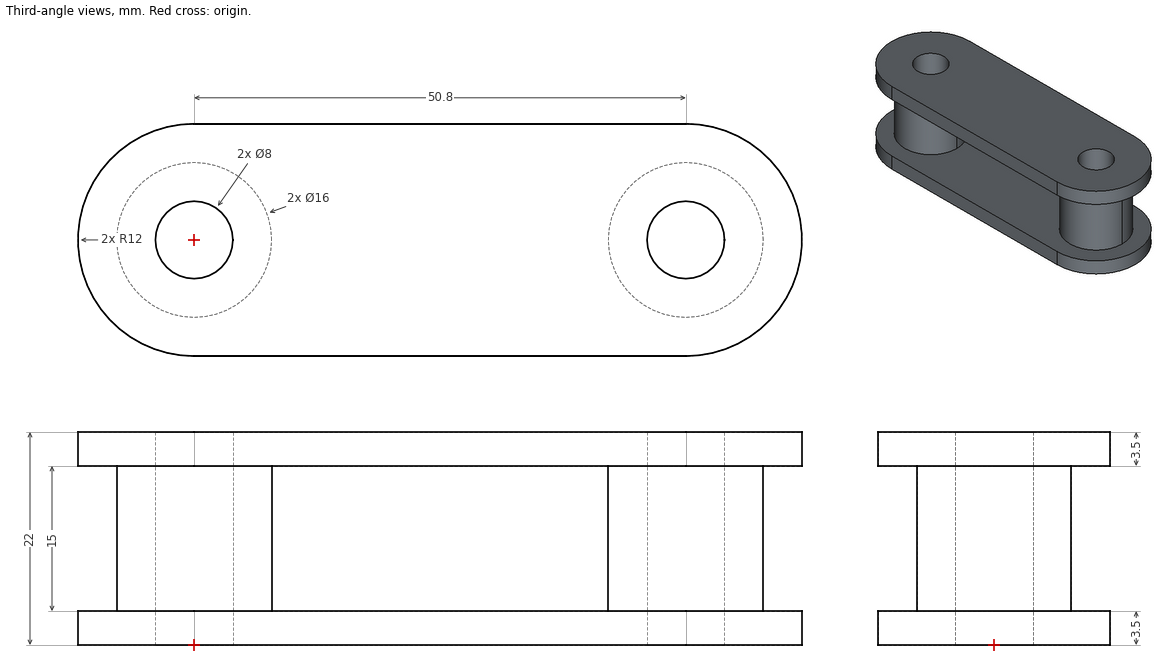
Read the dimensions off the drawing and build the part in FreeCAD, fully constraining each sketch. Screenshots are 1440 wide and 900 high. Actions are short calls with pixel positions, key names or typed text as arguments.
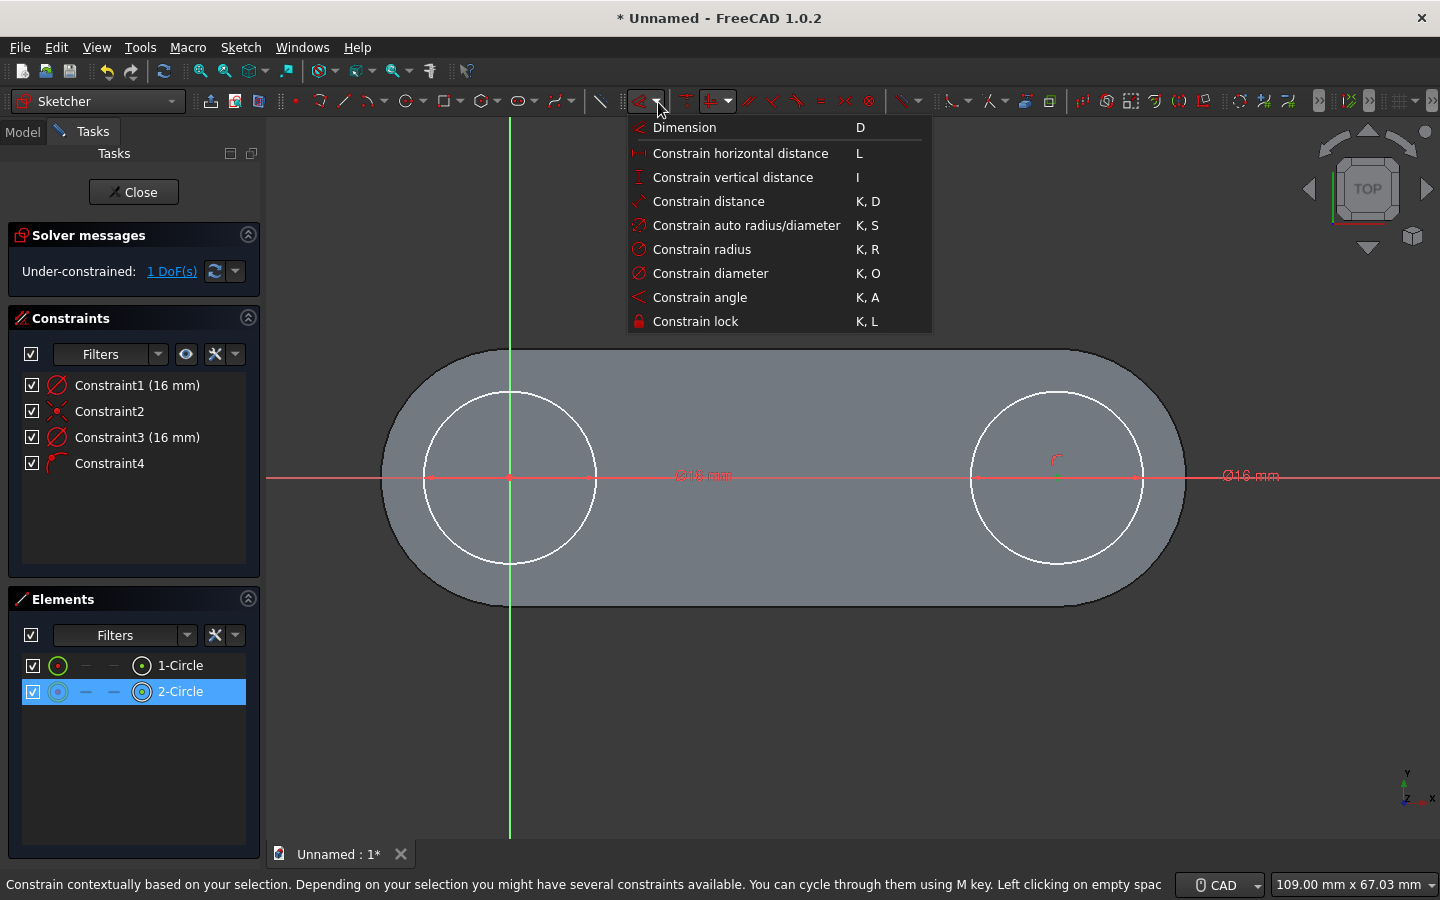
click(780, 153)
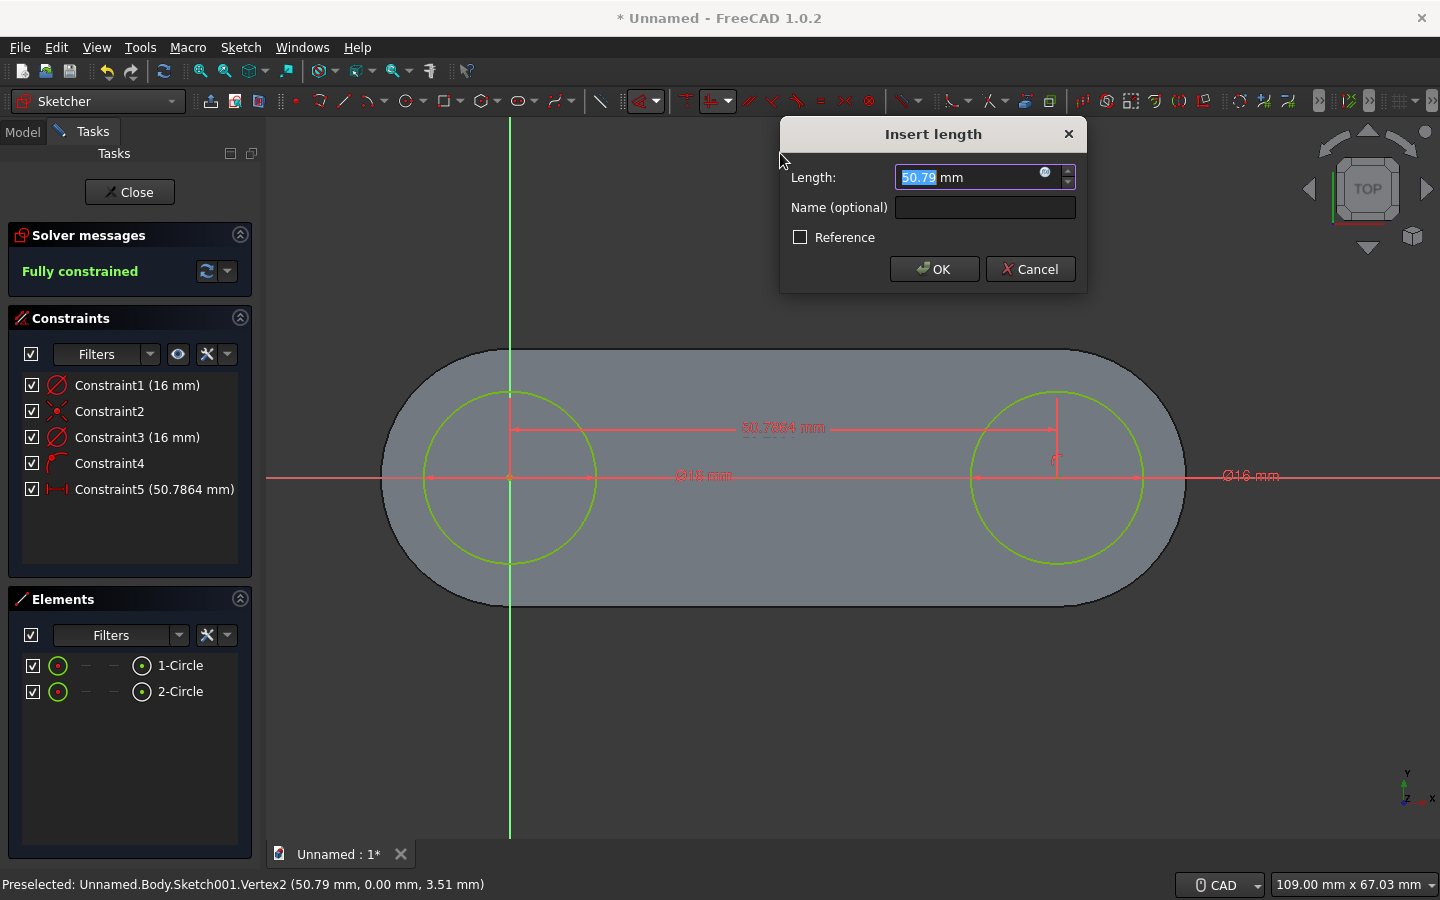
text(50.8)
key(Return)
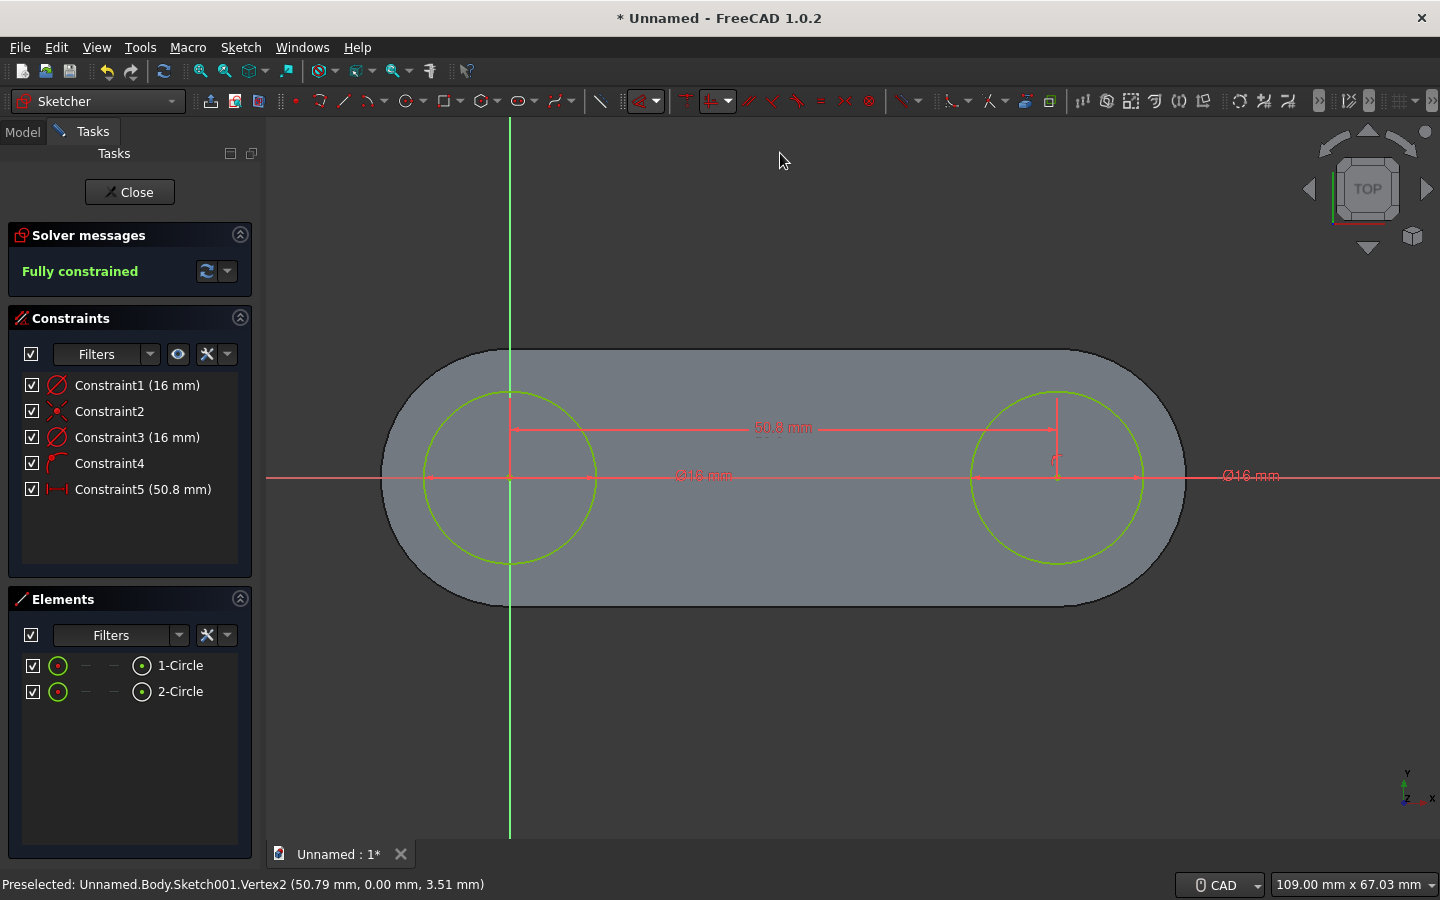
click(130, 192)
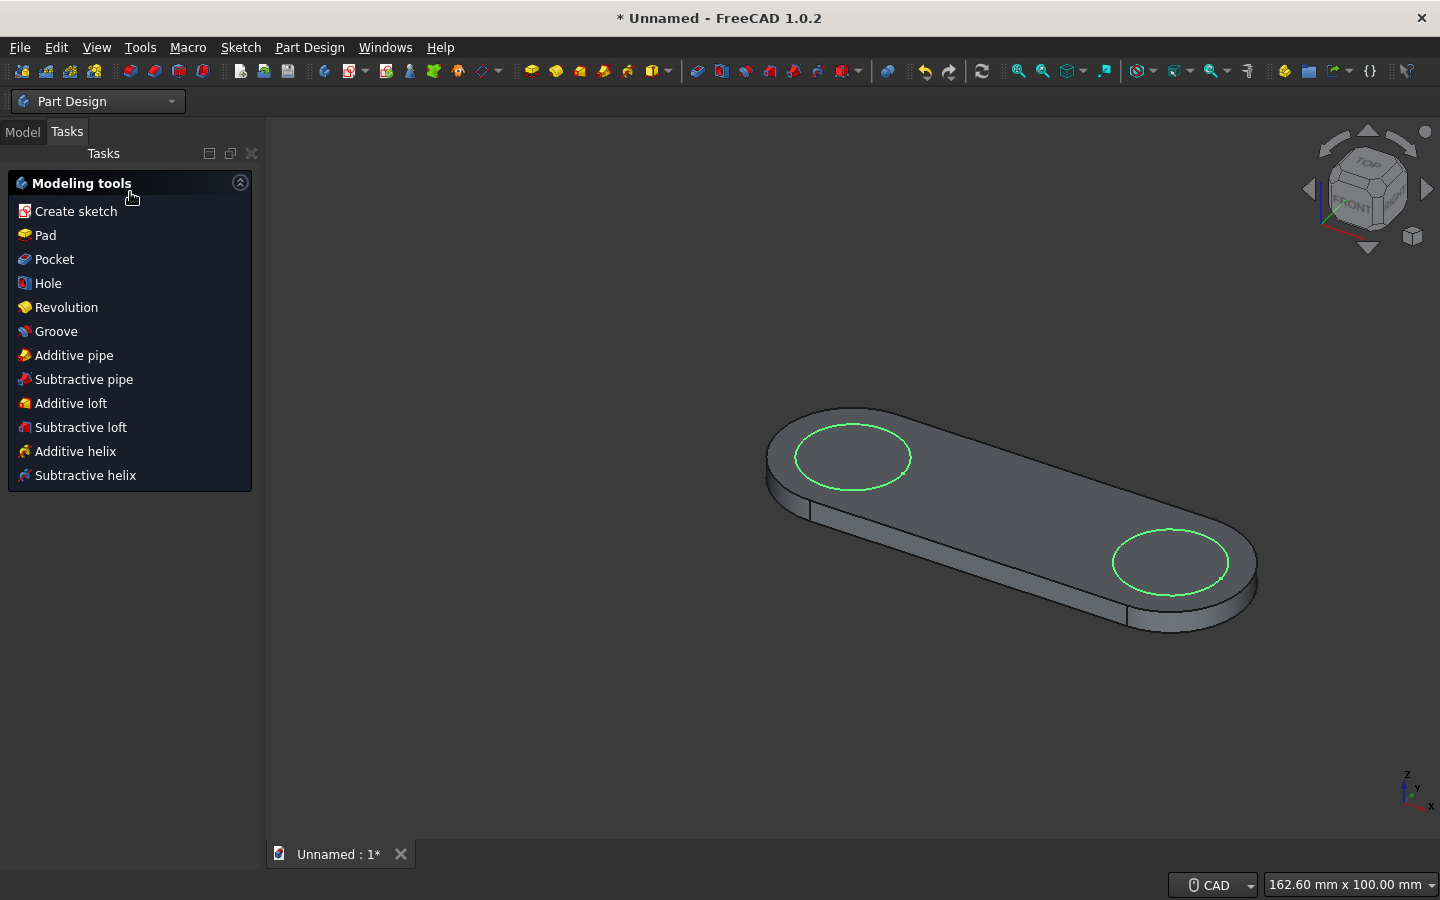
click(532, 72)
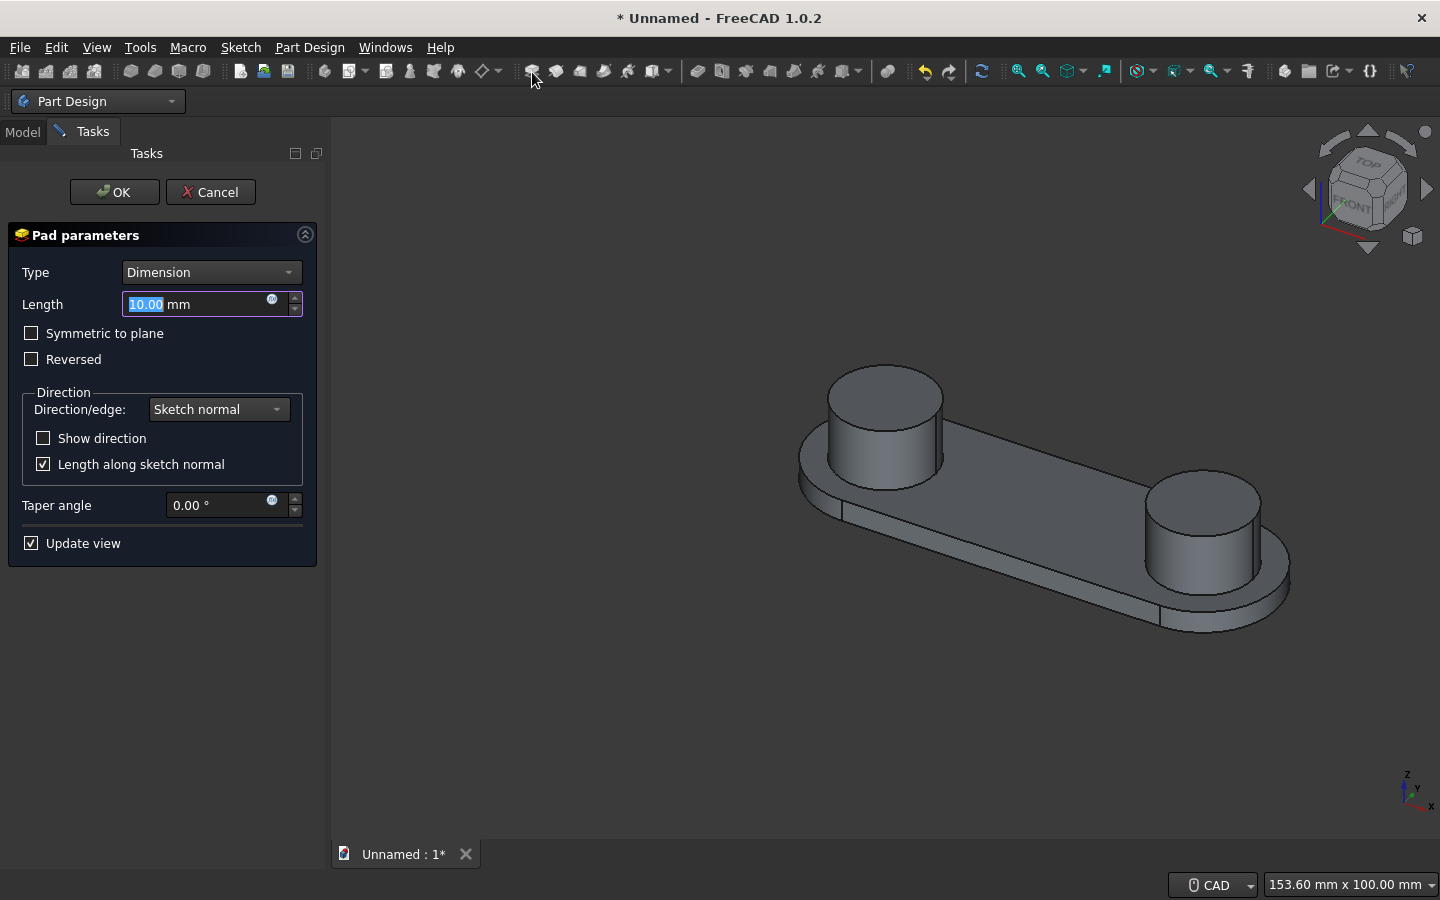
text(15)
key(Tab)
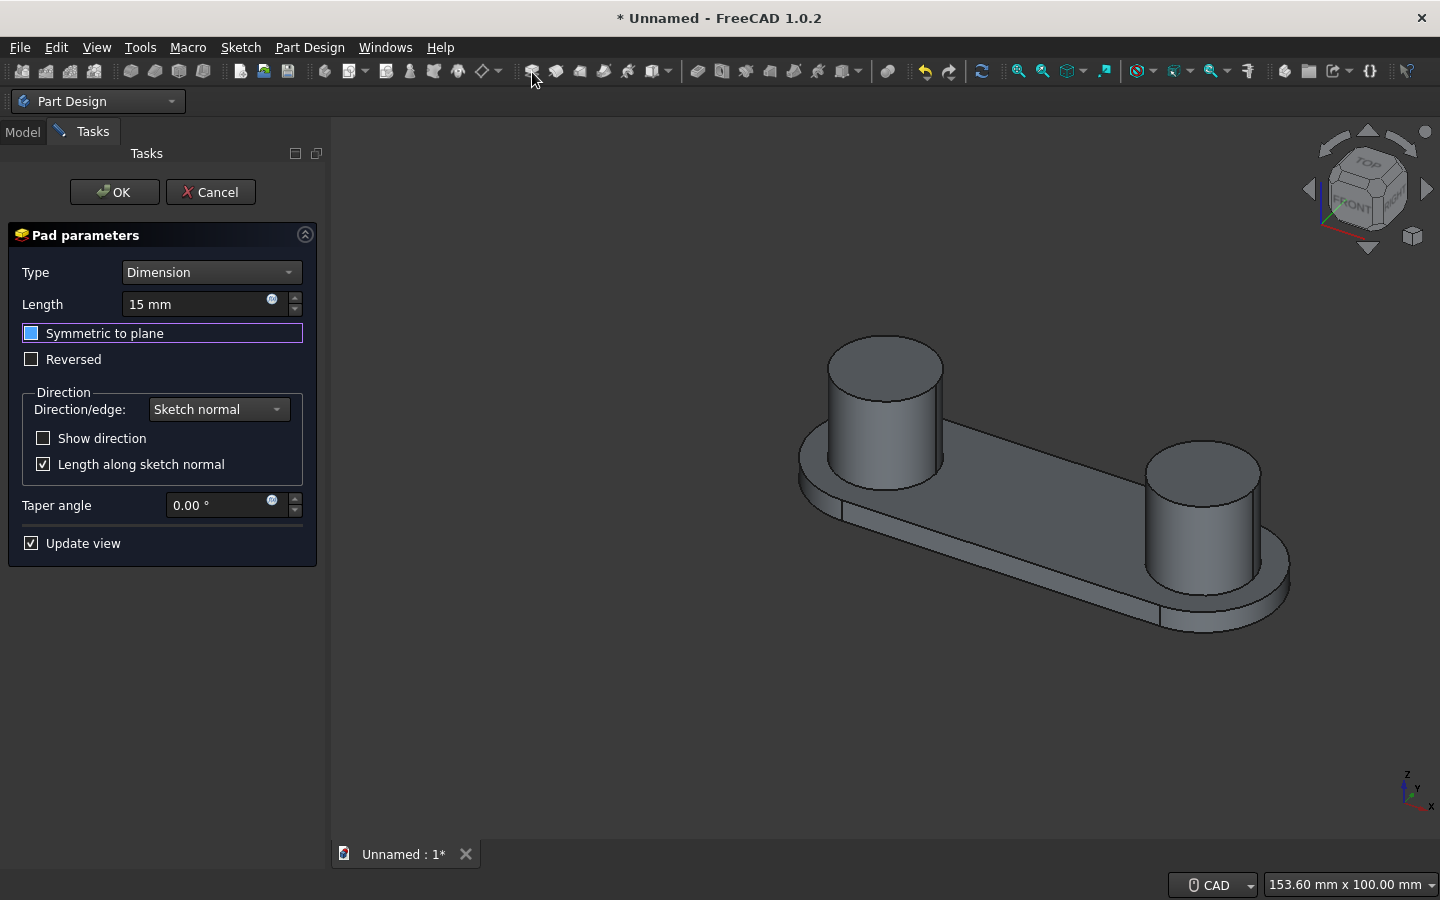
click(115, 192)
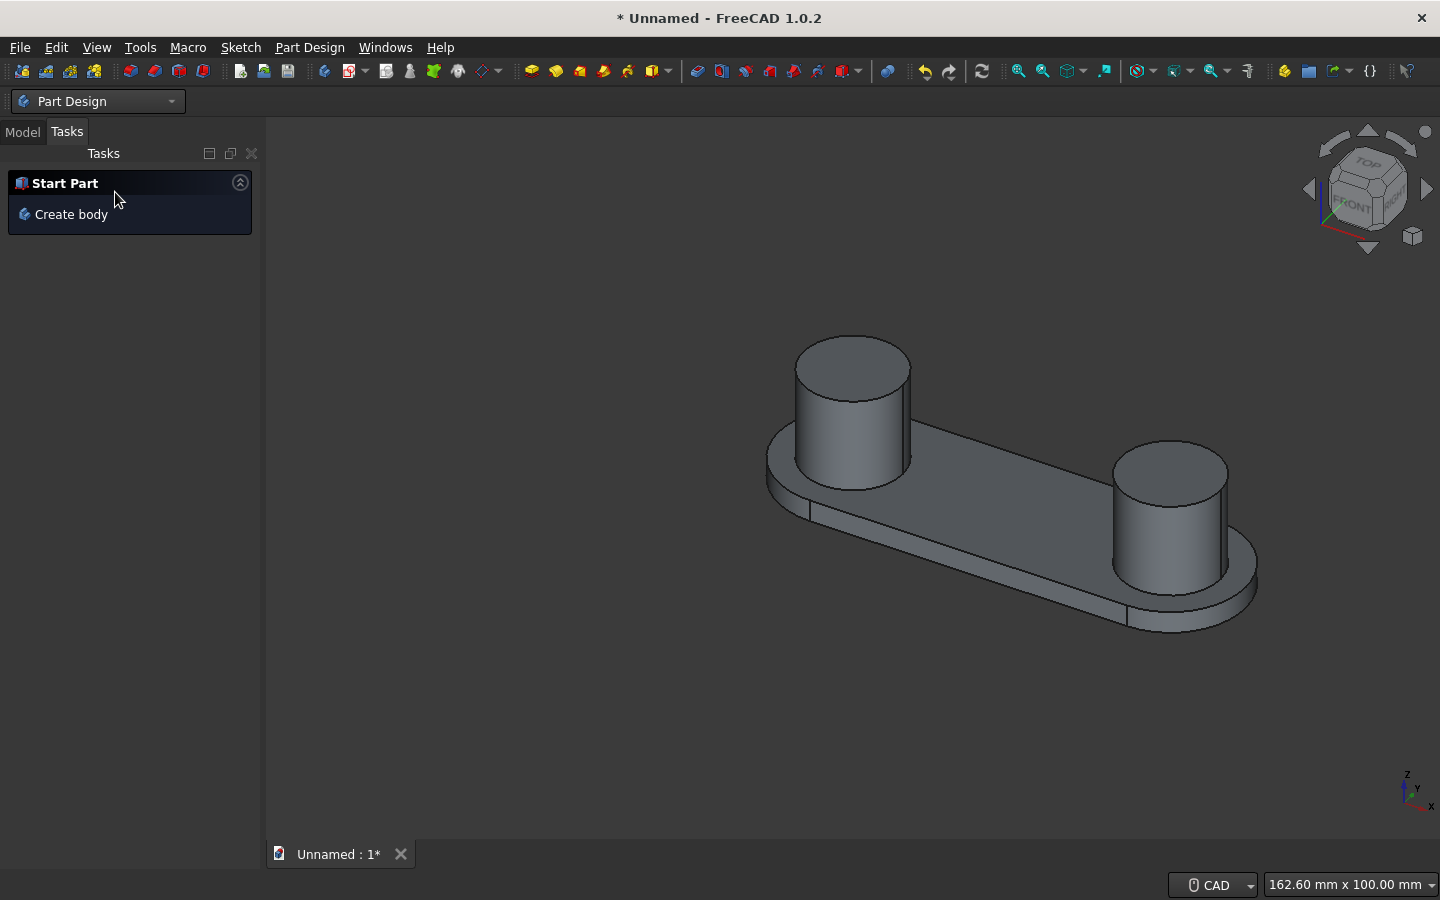
click(853, 368)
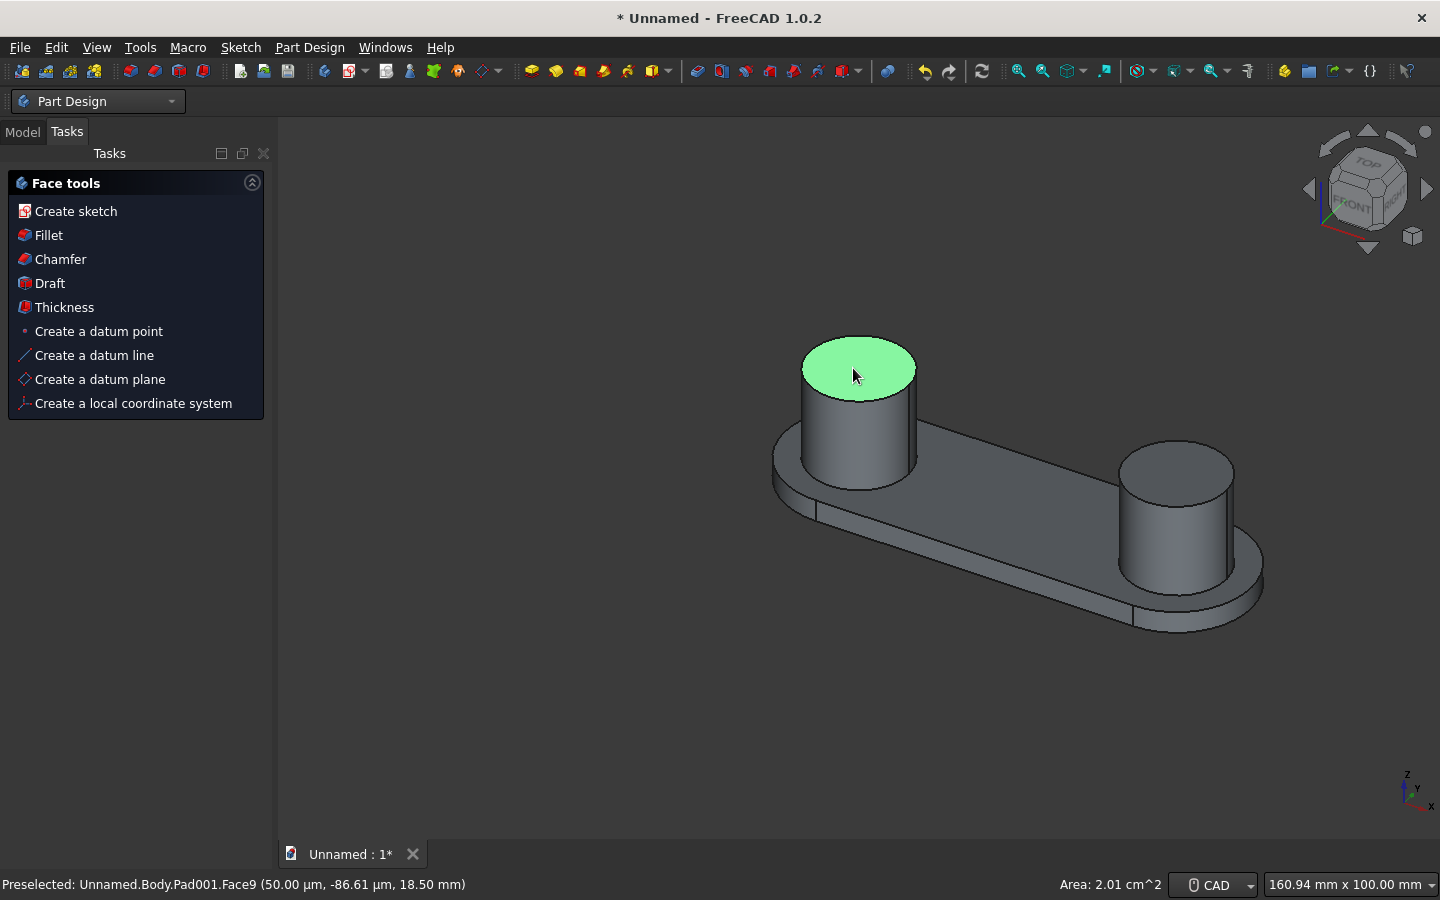
click(350, 72)